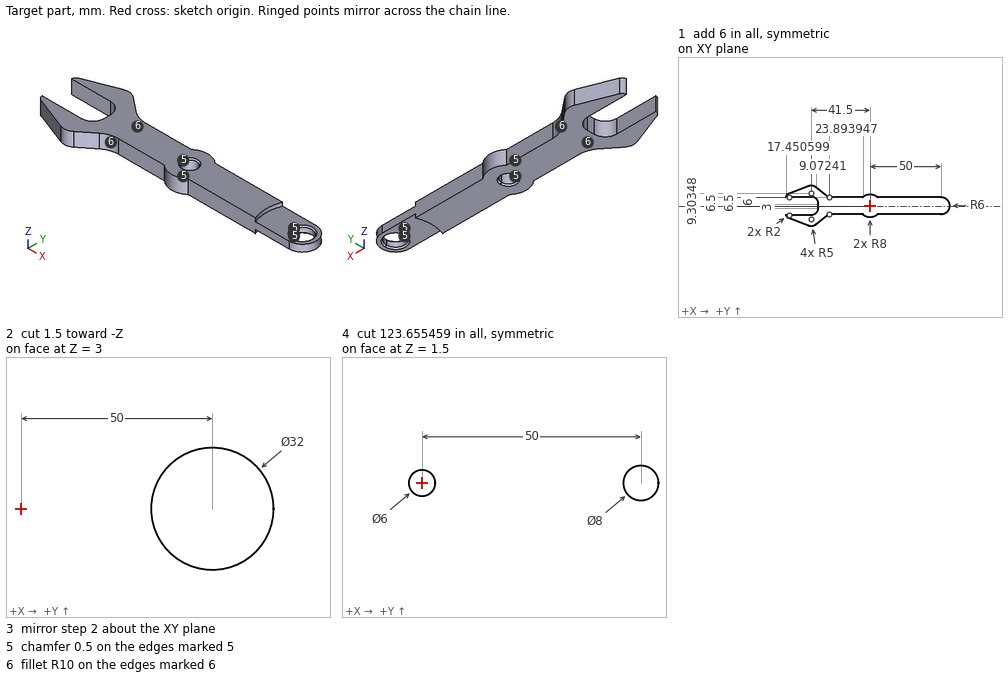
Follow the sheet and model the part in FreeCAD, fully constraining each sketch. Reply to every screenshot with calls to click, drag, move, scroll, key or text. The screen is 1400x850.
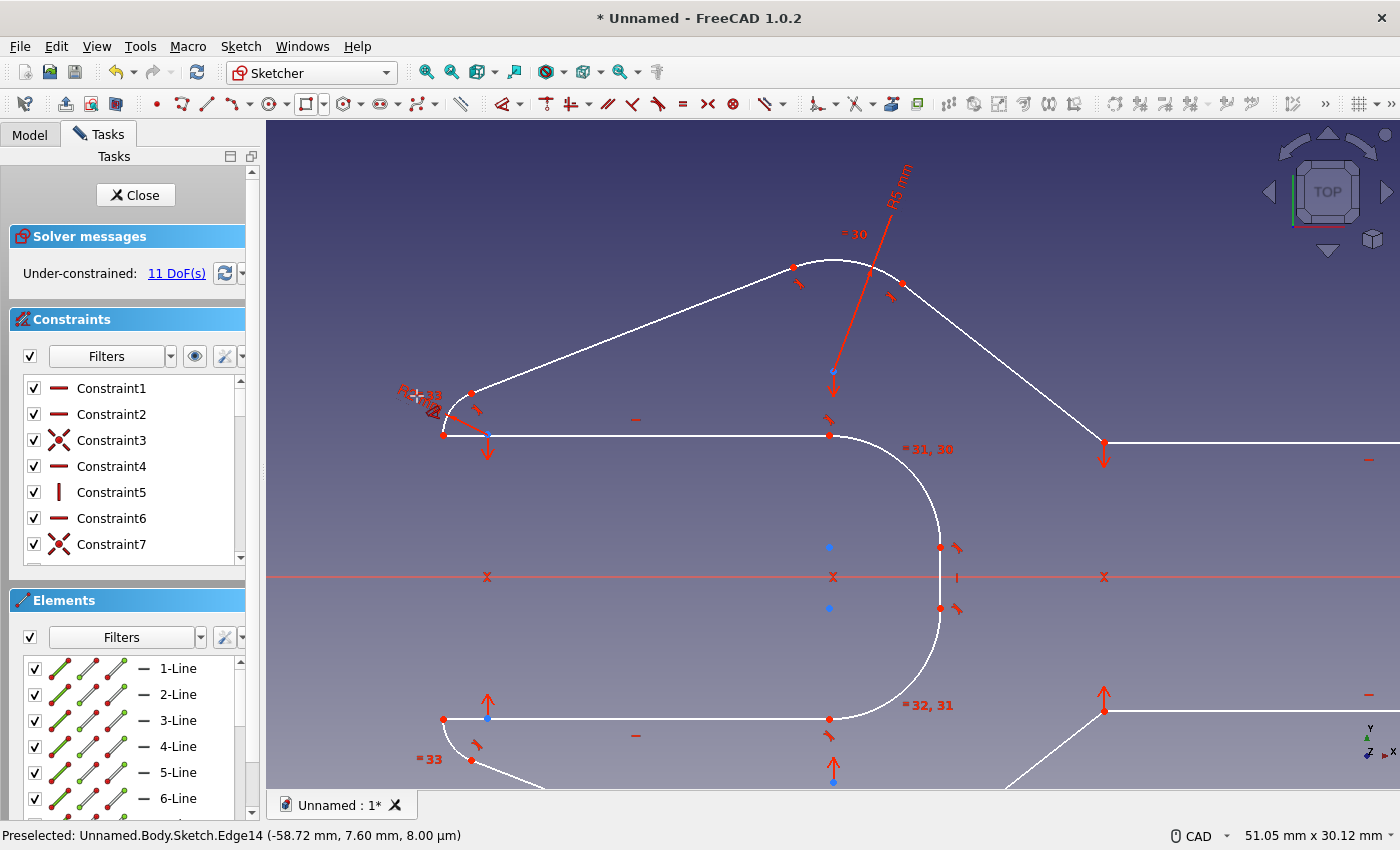
scroll(452, 414, down, 7)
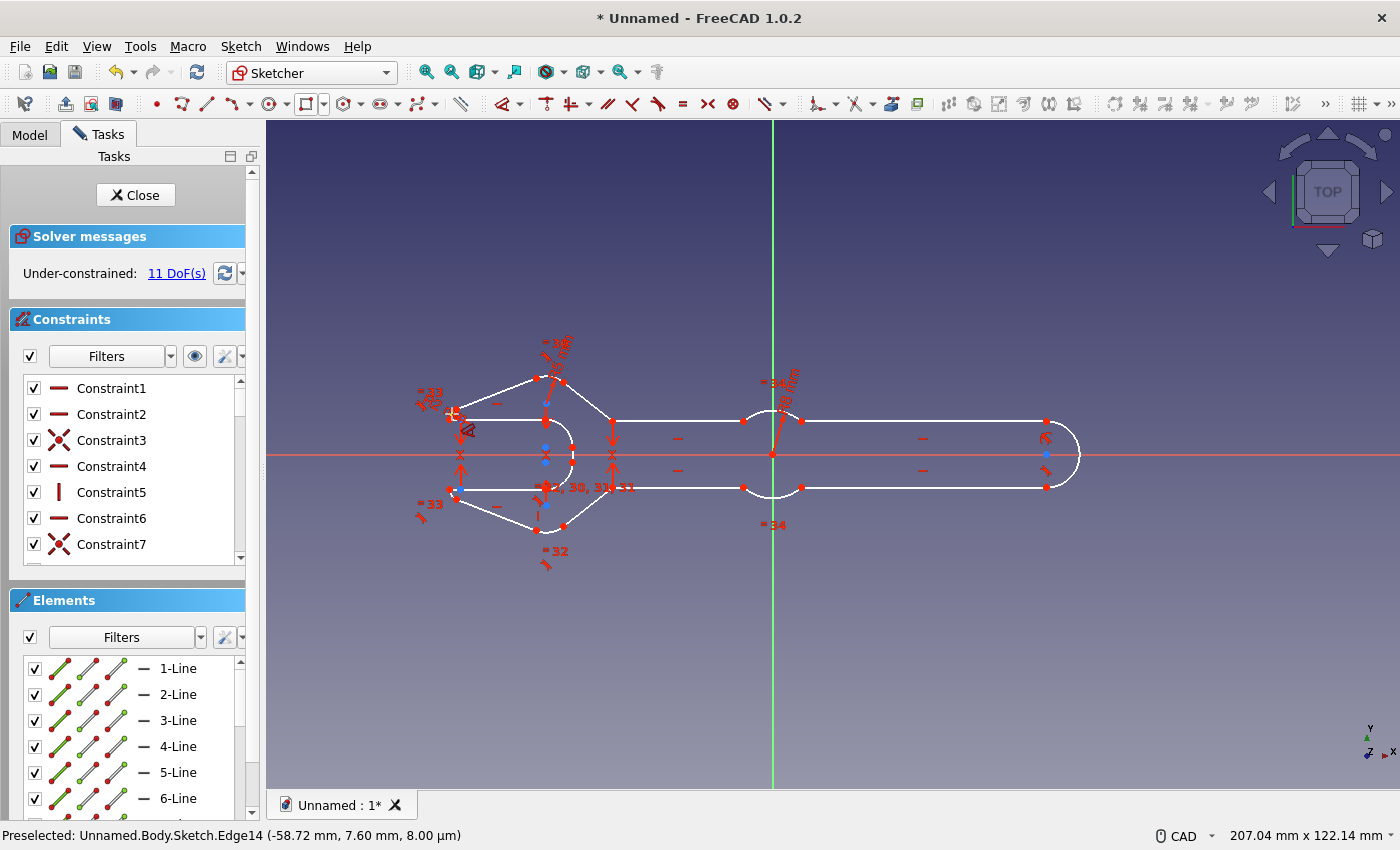
click(1073, 474)
click(1099, 493)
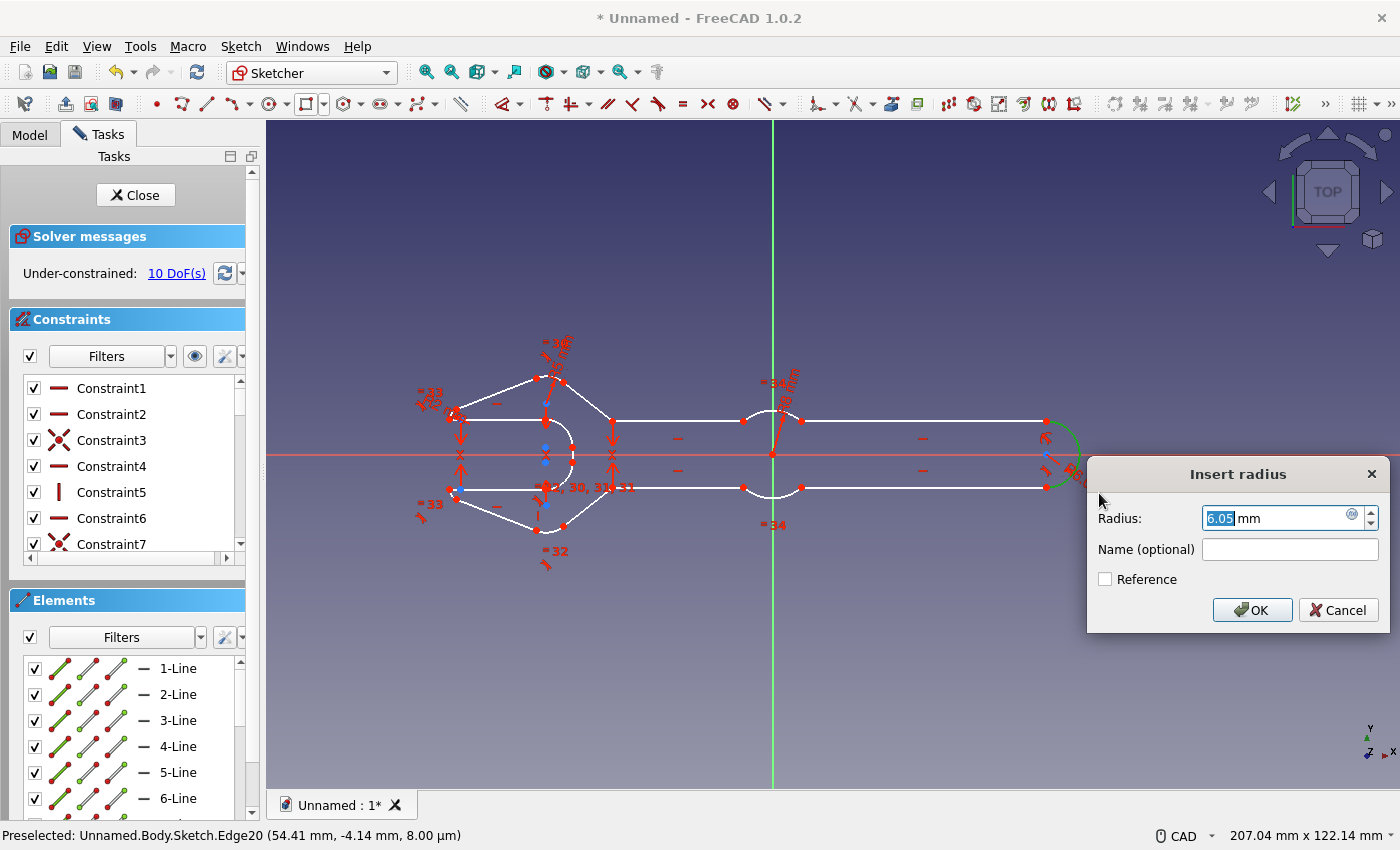
text(6)
key(Return)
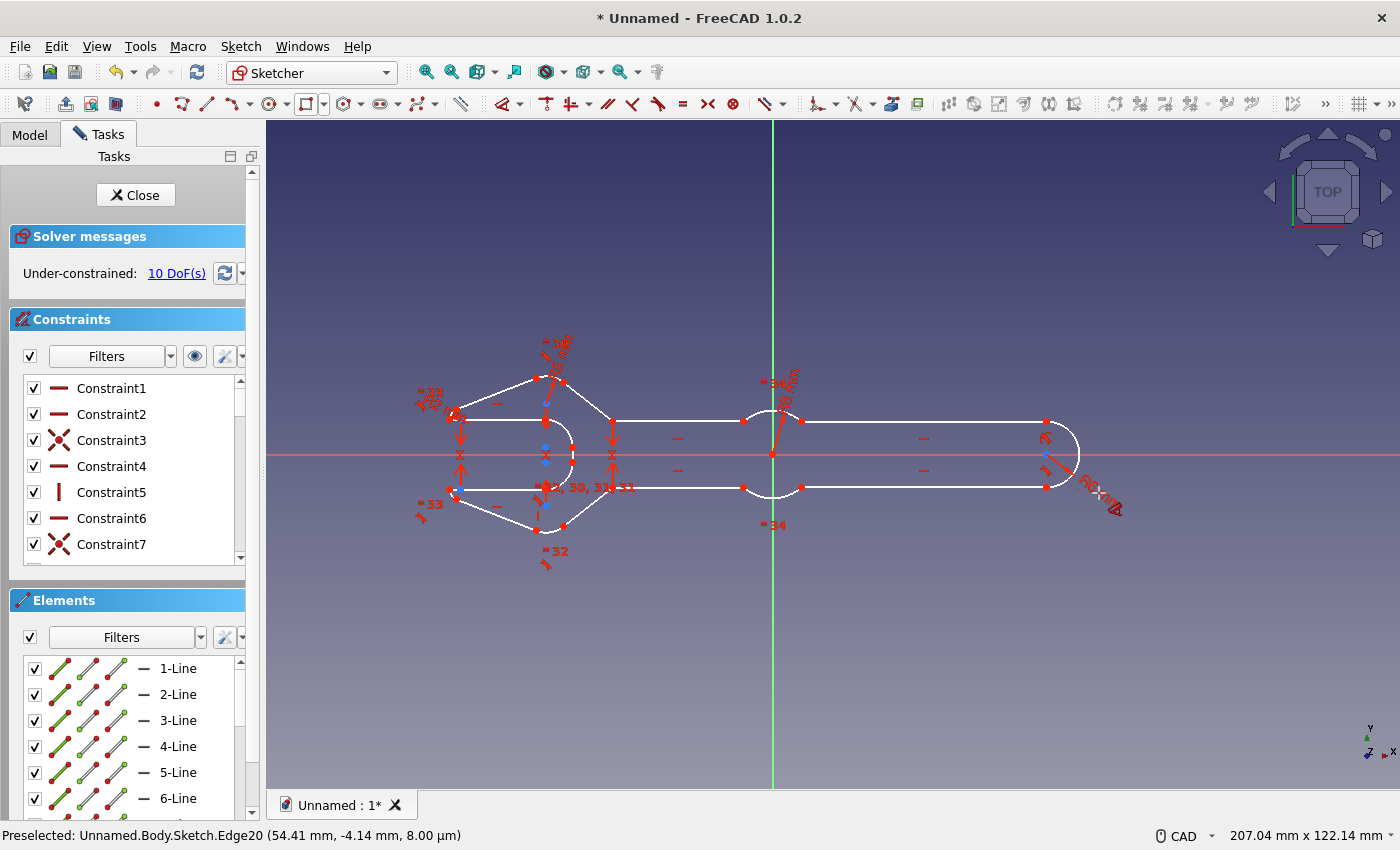
scroll(573, 455, up, 5)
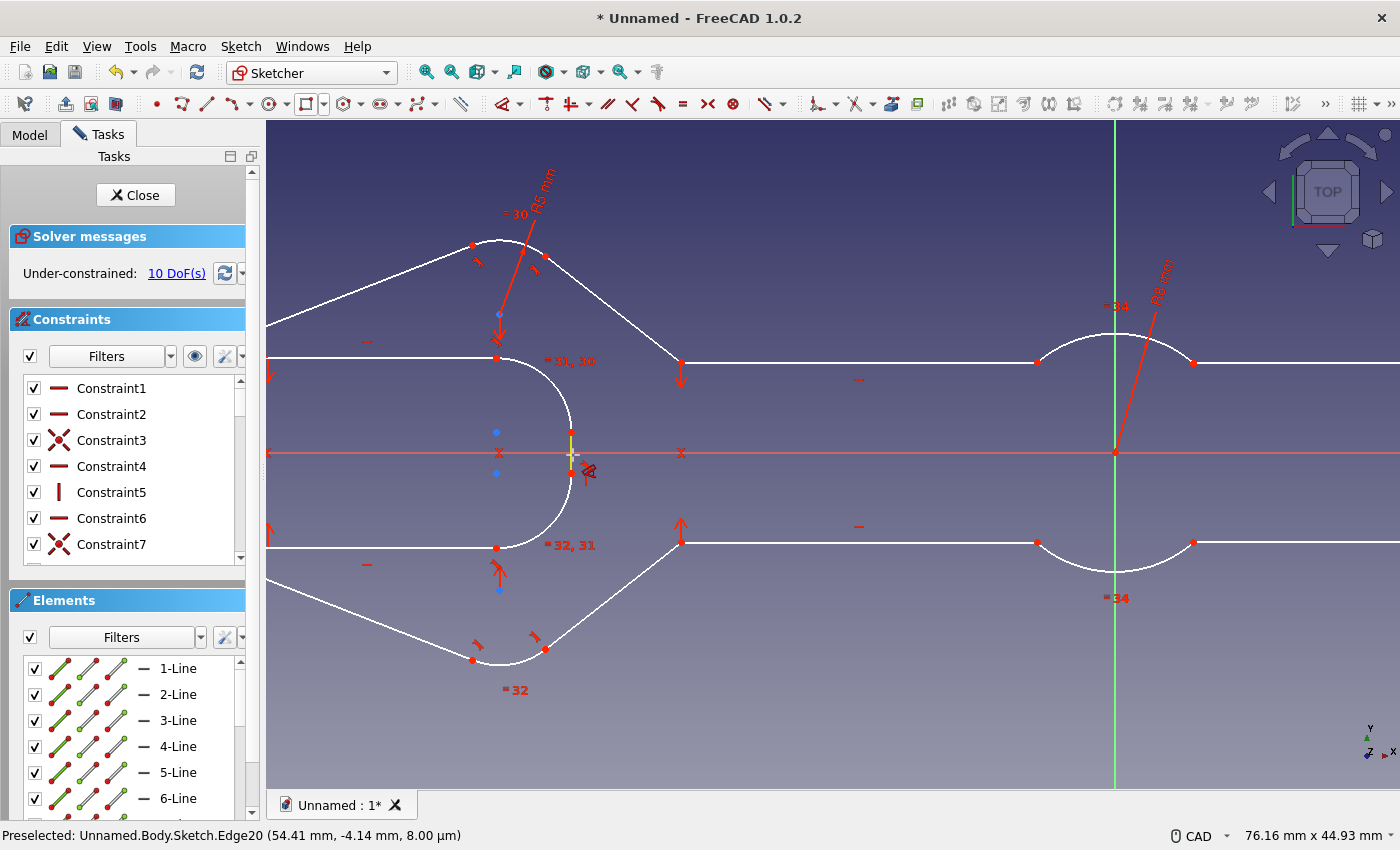
click(571, 453)
click(537, 439)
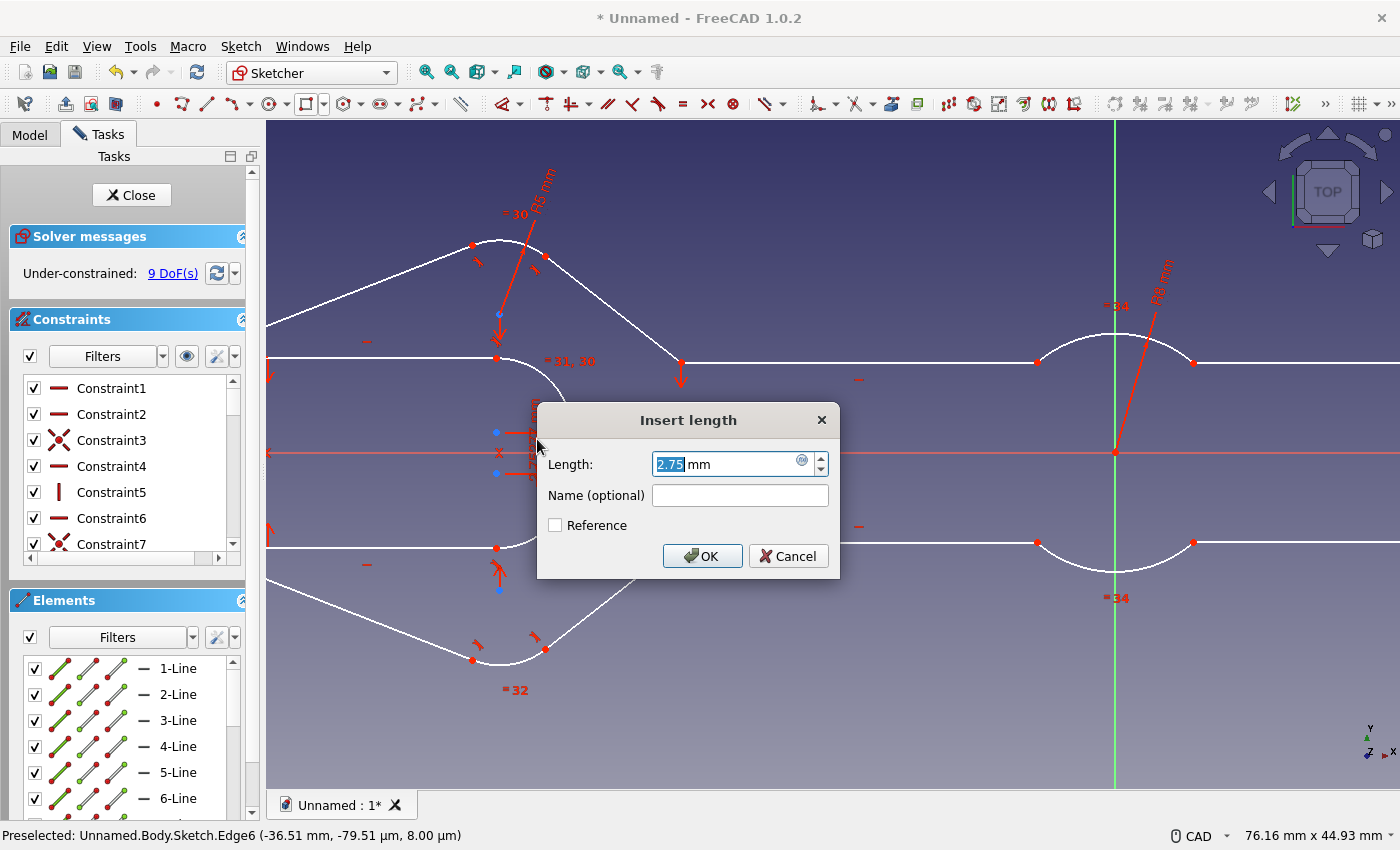
text(3)
key(Return)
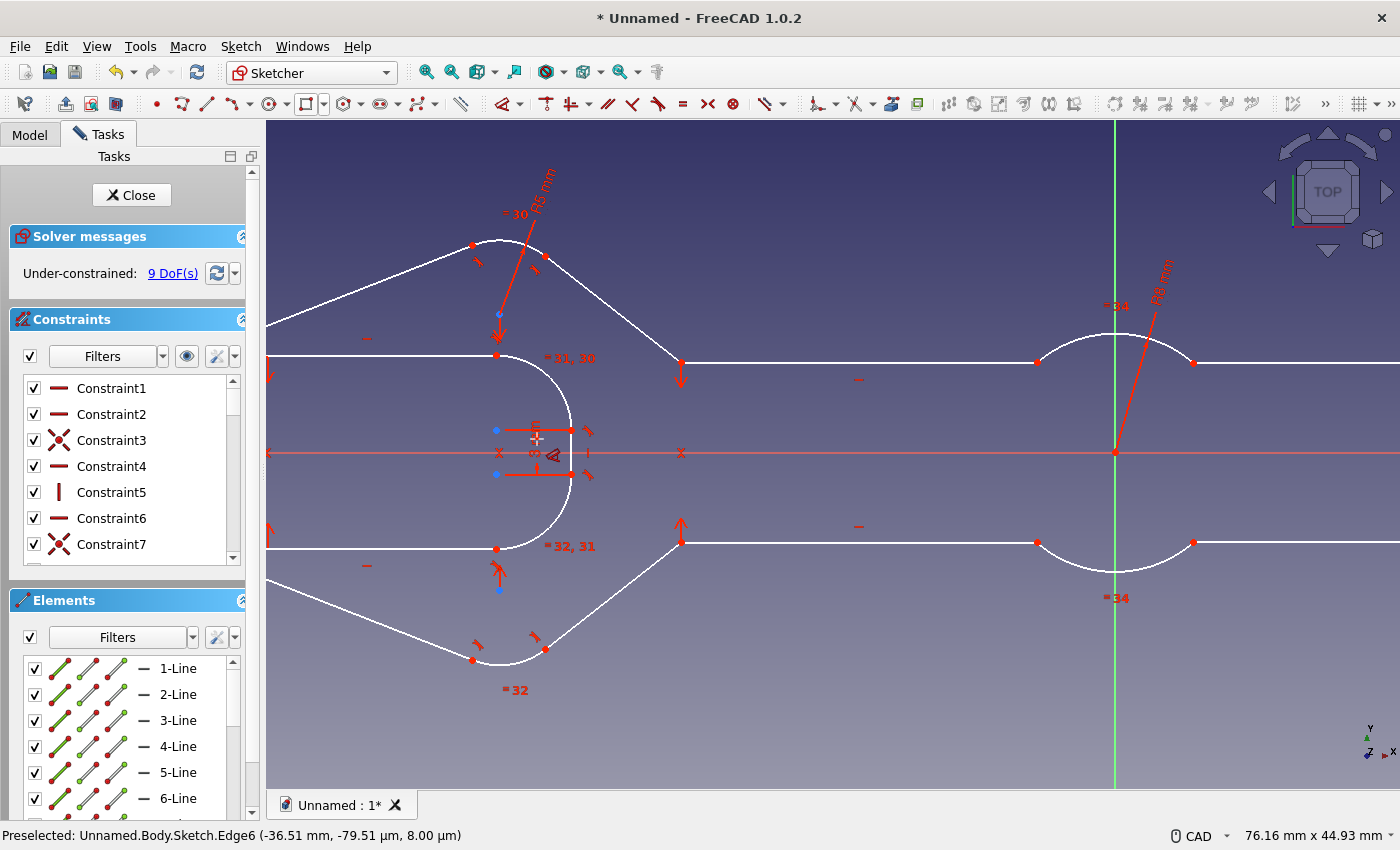
click(1037, 363)
click(1003, 408)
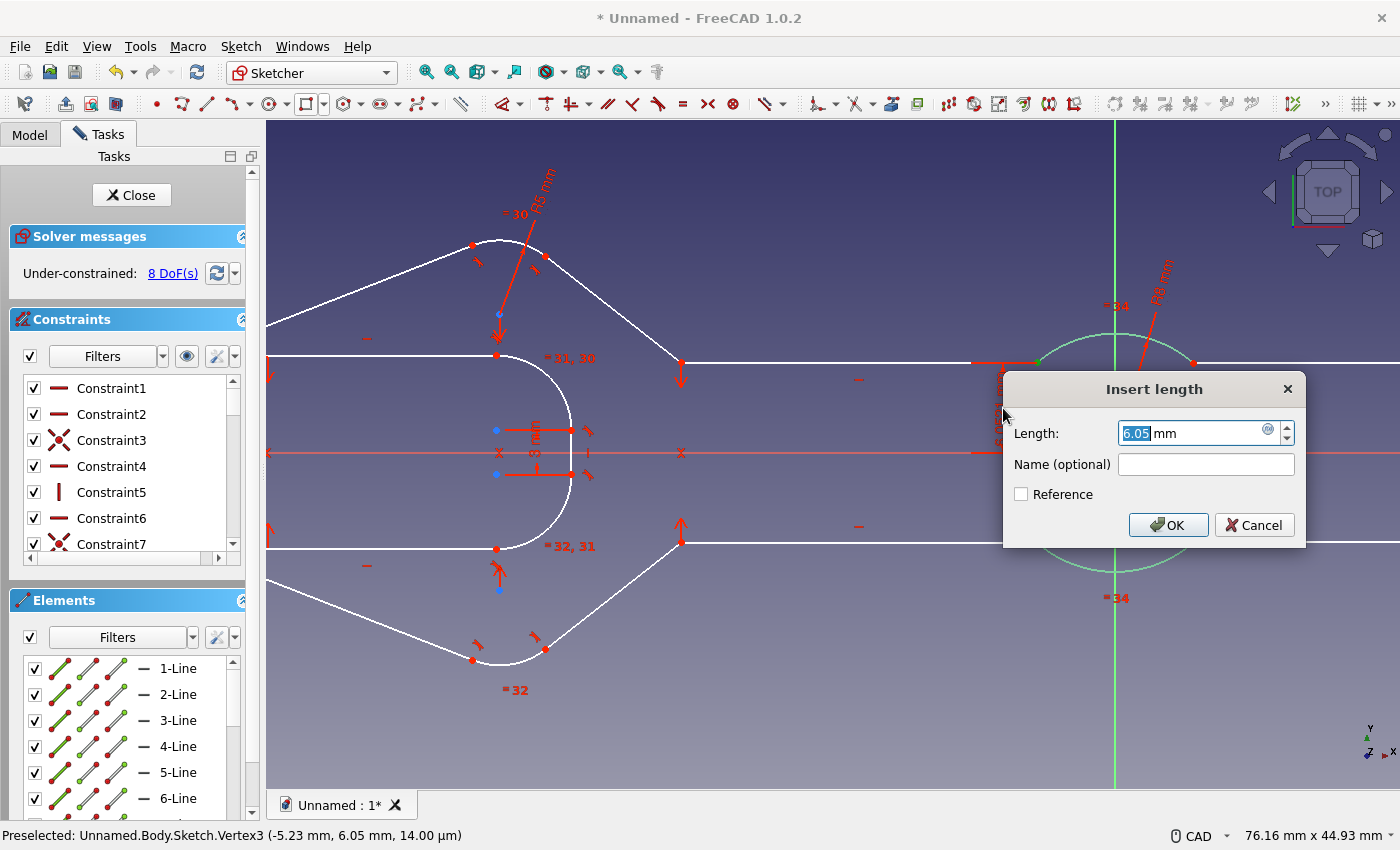
text(6)
key(Return)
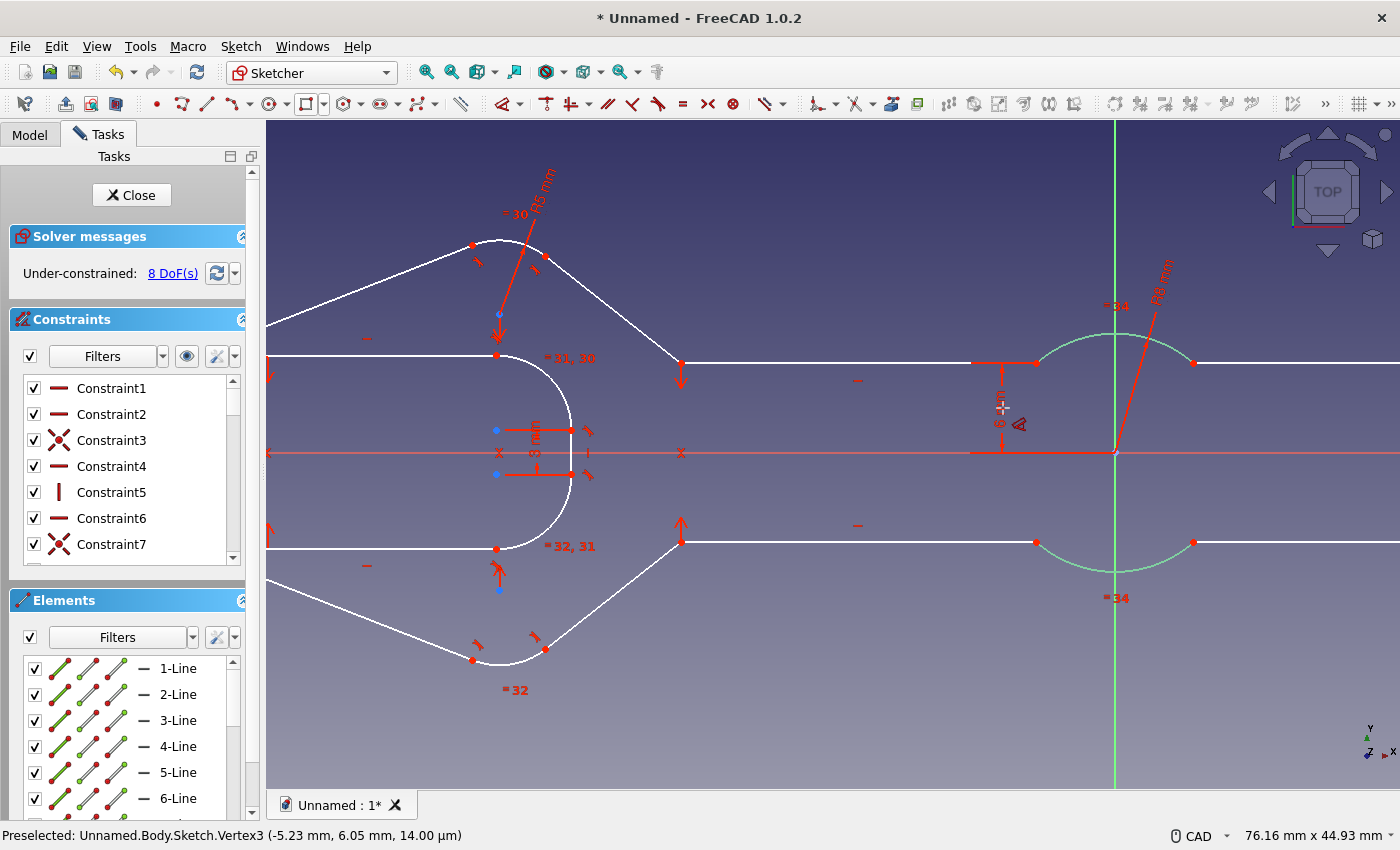
scroll(573, 455, down, 5)